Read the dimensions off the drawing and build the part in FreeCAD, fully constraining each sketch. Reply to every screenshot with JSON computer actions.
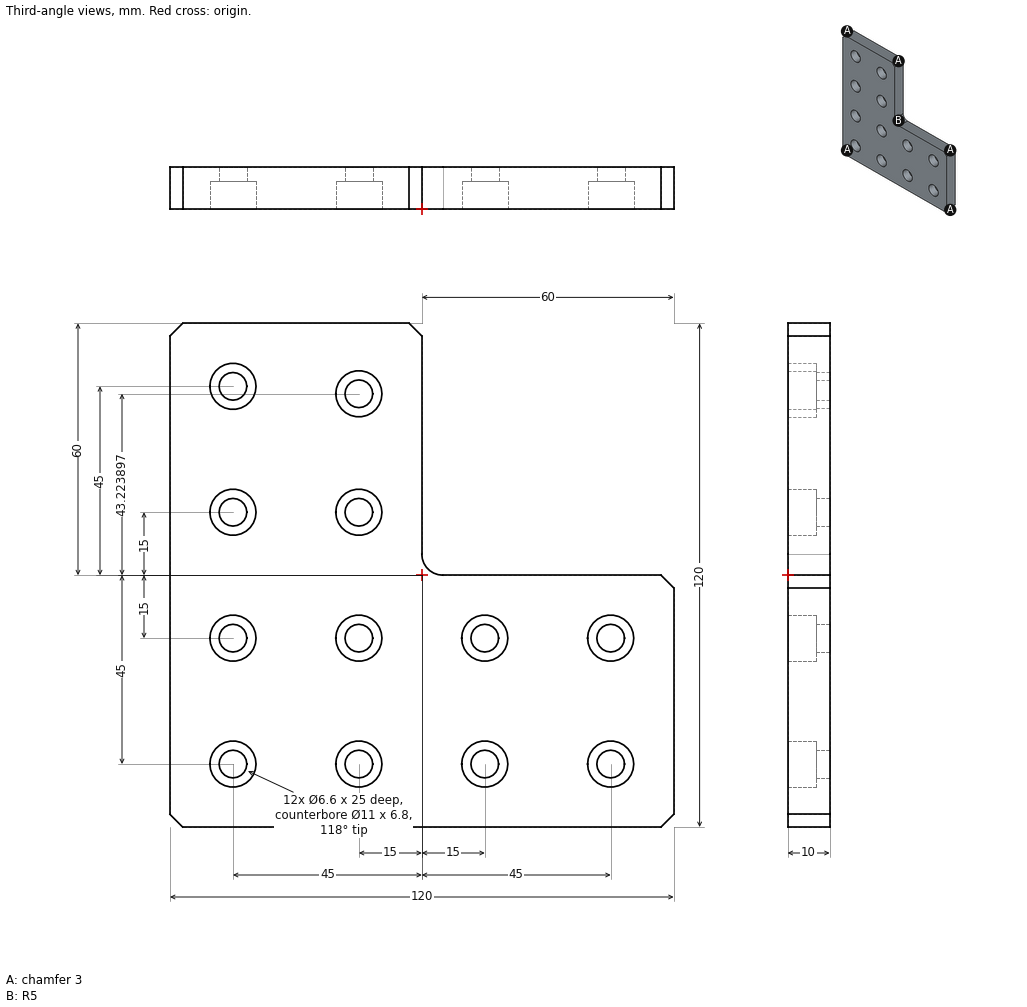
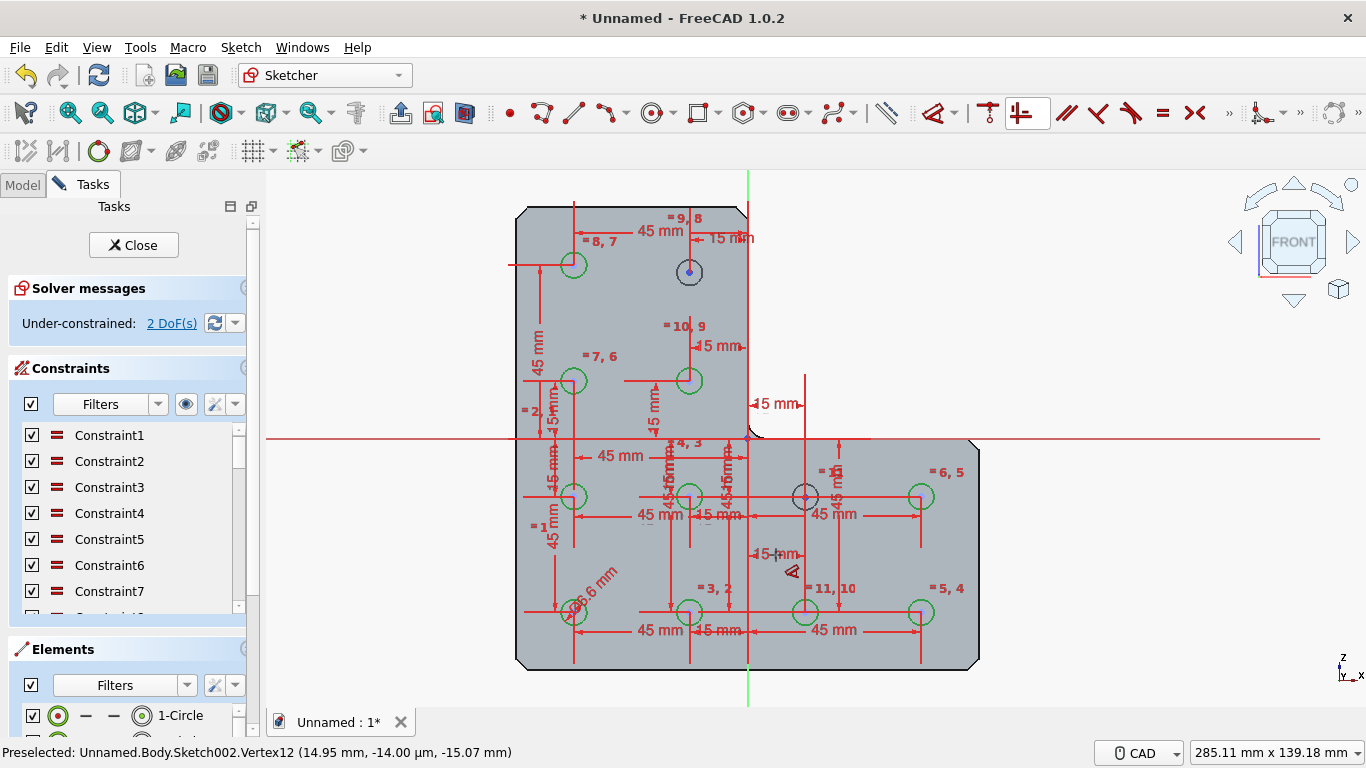
{"action": "left_click", "coordinate": [805, 497]}
{"action": "left_click", "coordinate": [839, 455]}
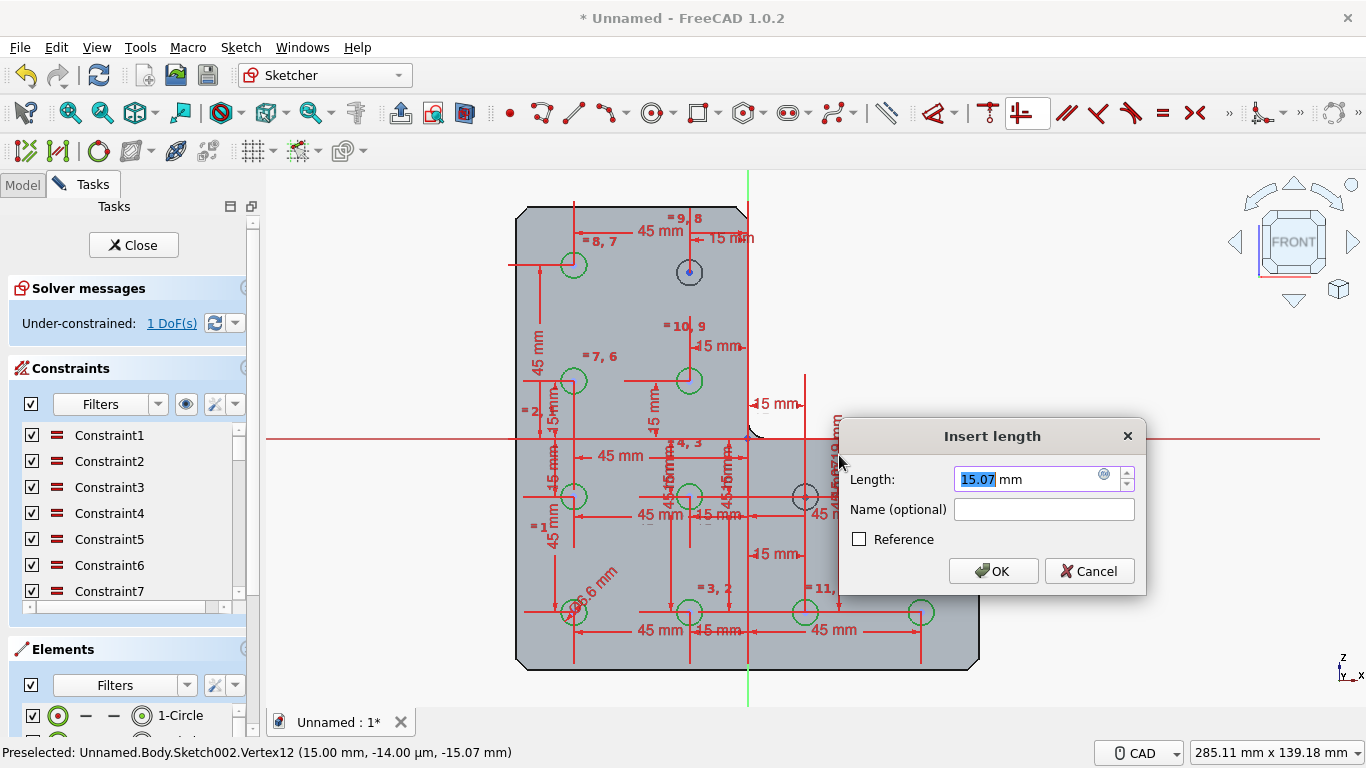
{"action": "type", "text": "15"}
{"action": "key", "text": "Return"}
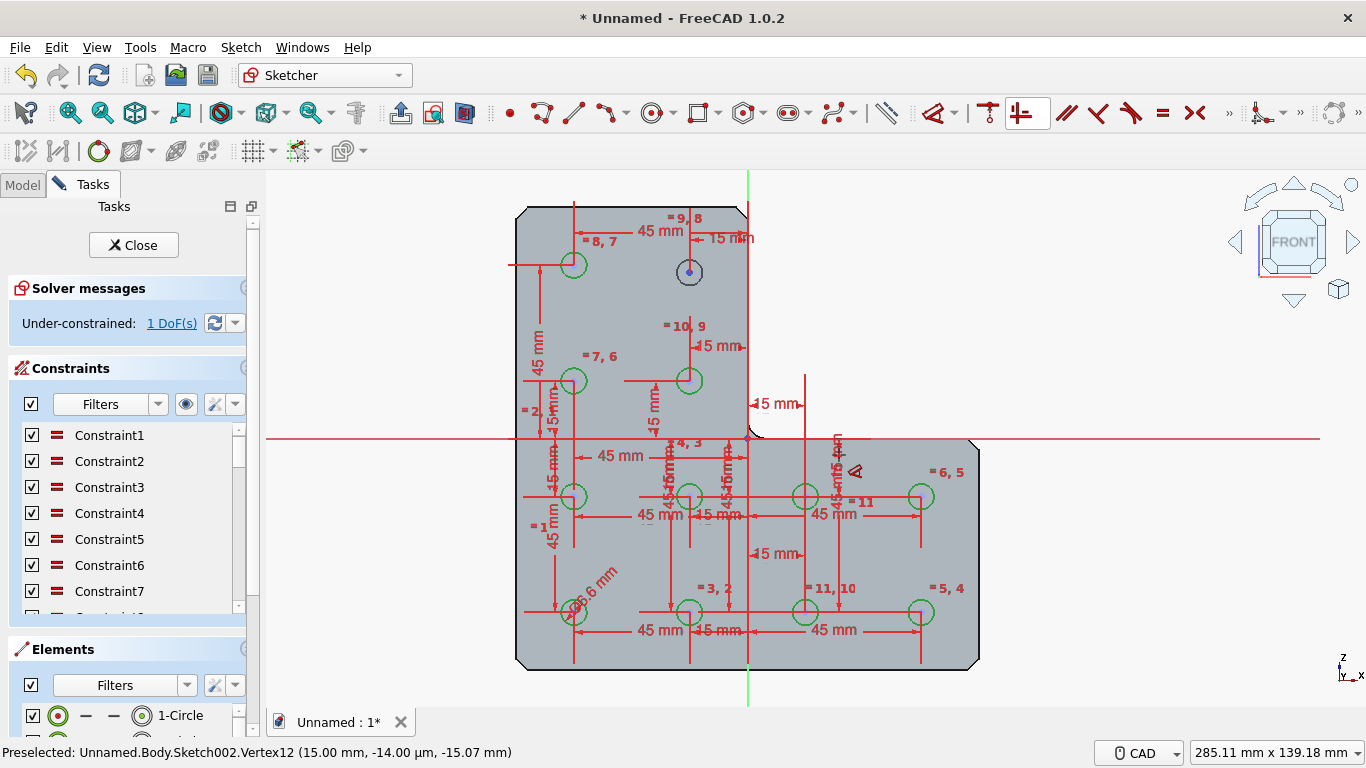
{"action": "left_click", "coordinate": [690, 273]}
{"action": "left_click", "coordinate": [656, 318]}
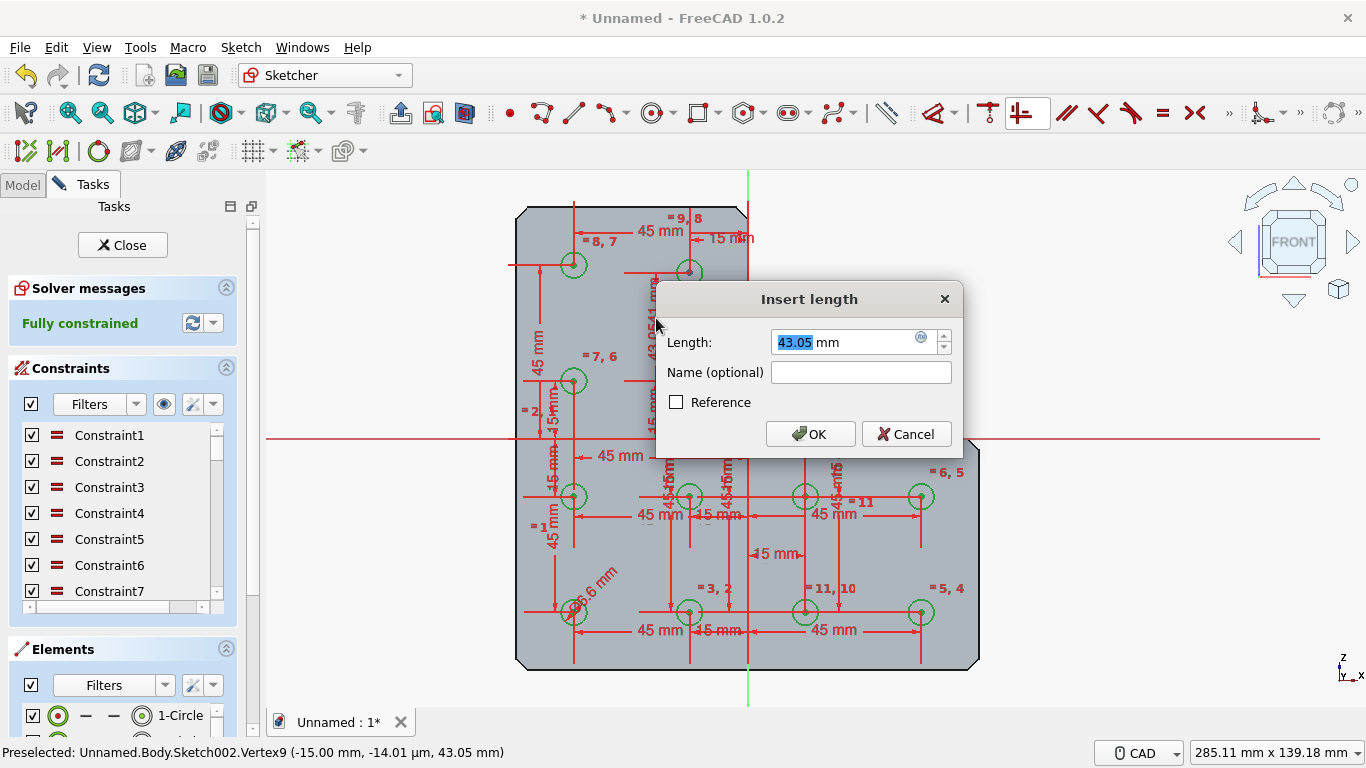
{"action": "type", "text": "43.223897"}
{"action": "key", "text": "Return"}
{"action": "key", "text": "Escape"}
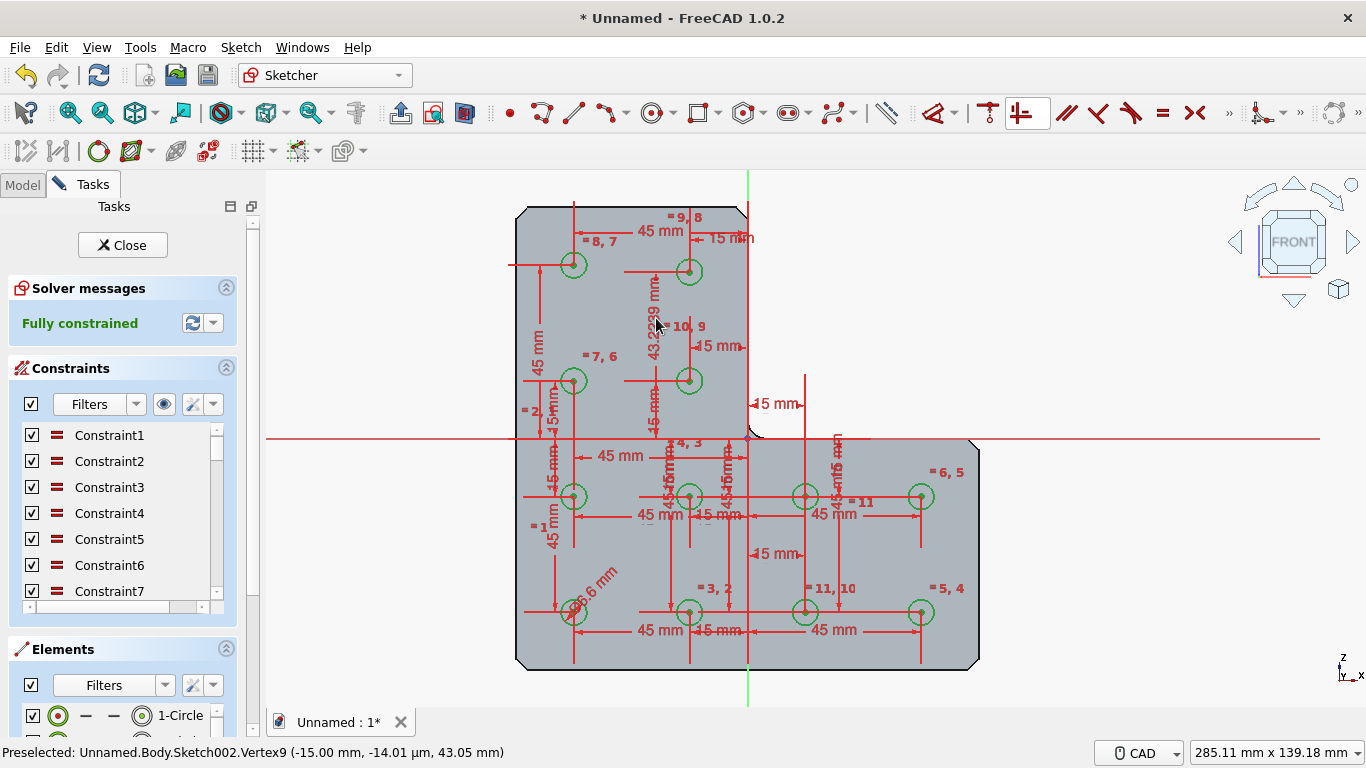
{"action": "left_click", "coordinate": [123, 245]}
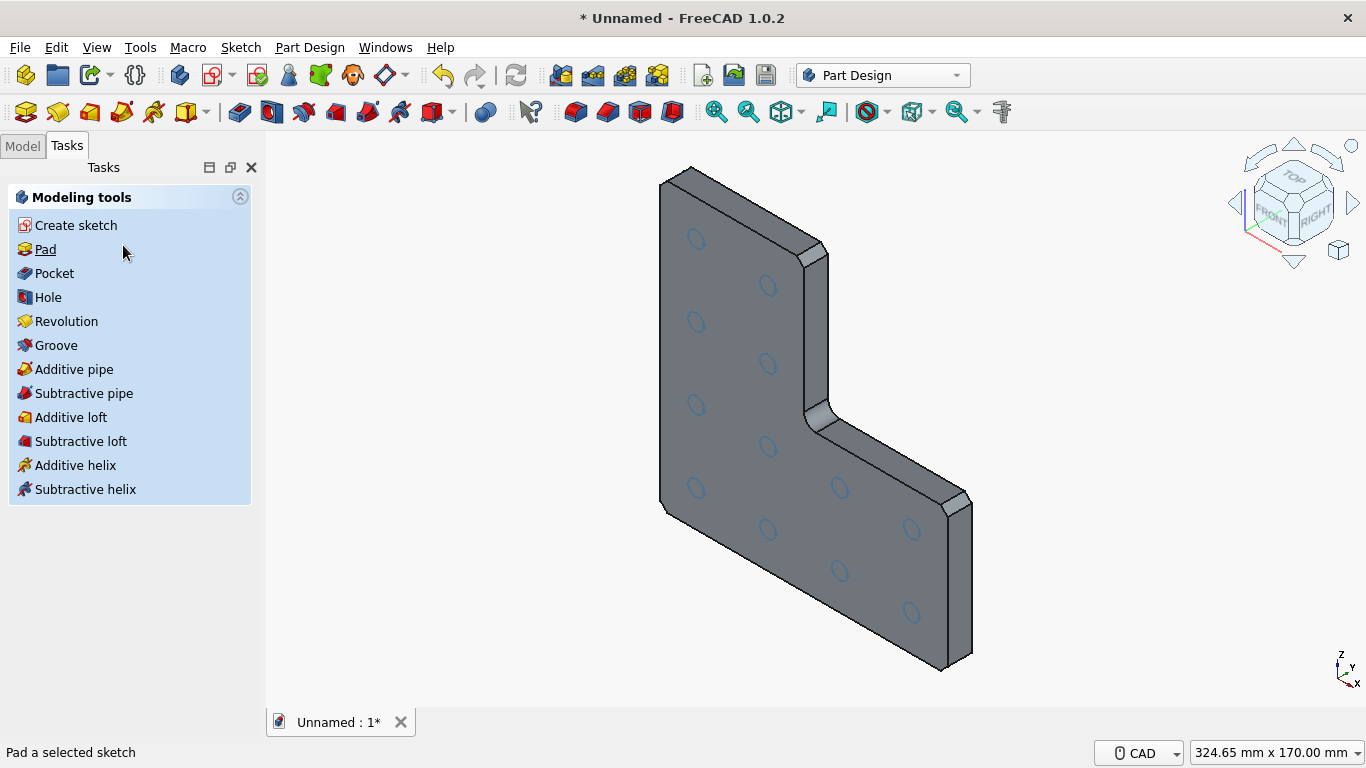
{"action": "left_click", "coordinate": [272, 112]}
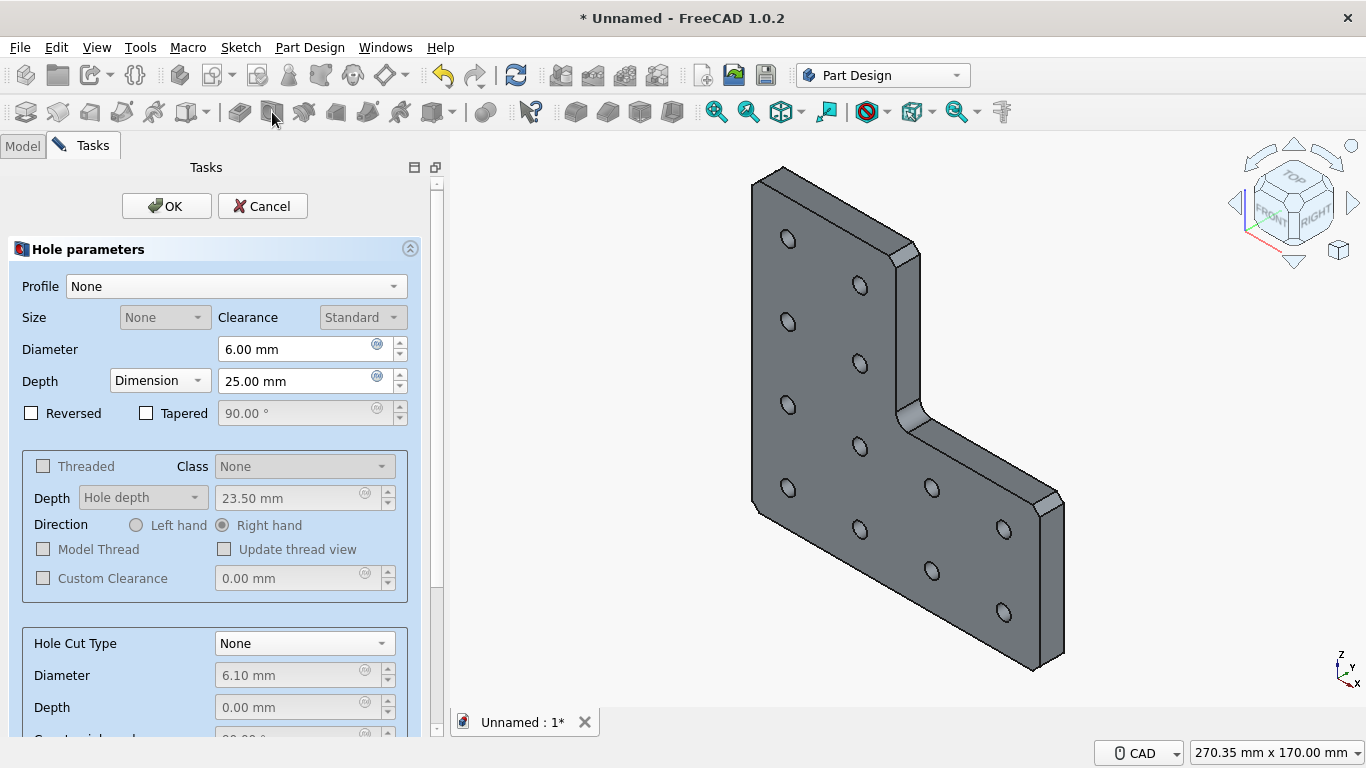
{"action": "triple_click", "coordinate": [305, 349]}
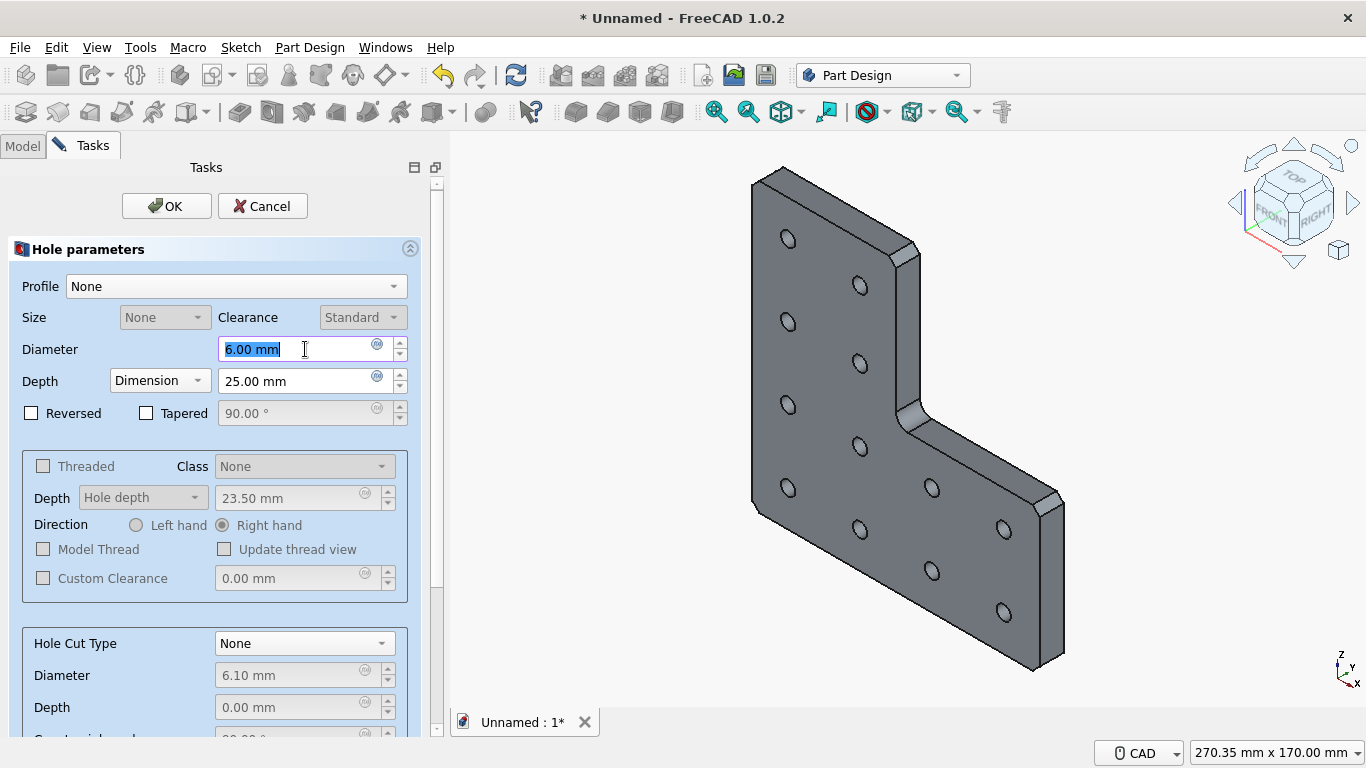
{"action": "type", "text": "6.6"}
{"action": "key", "text": "Tab"}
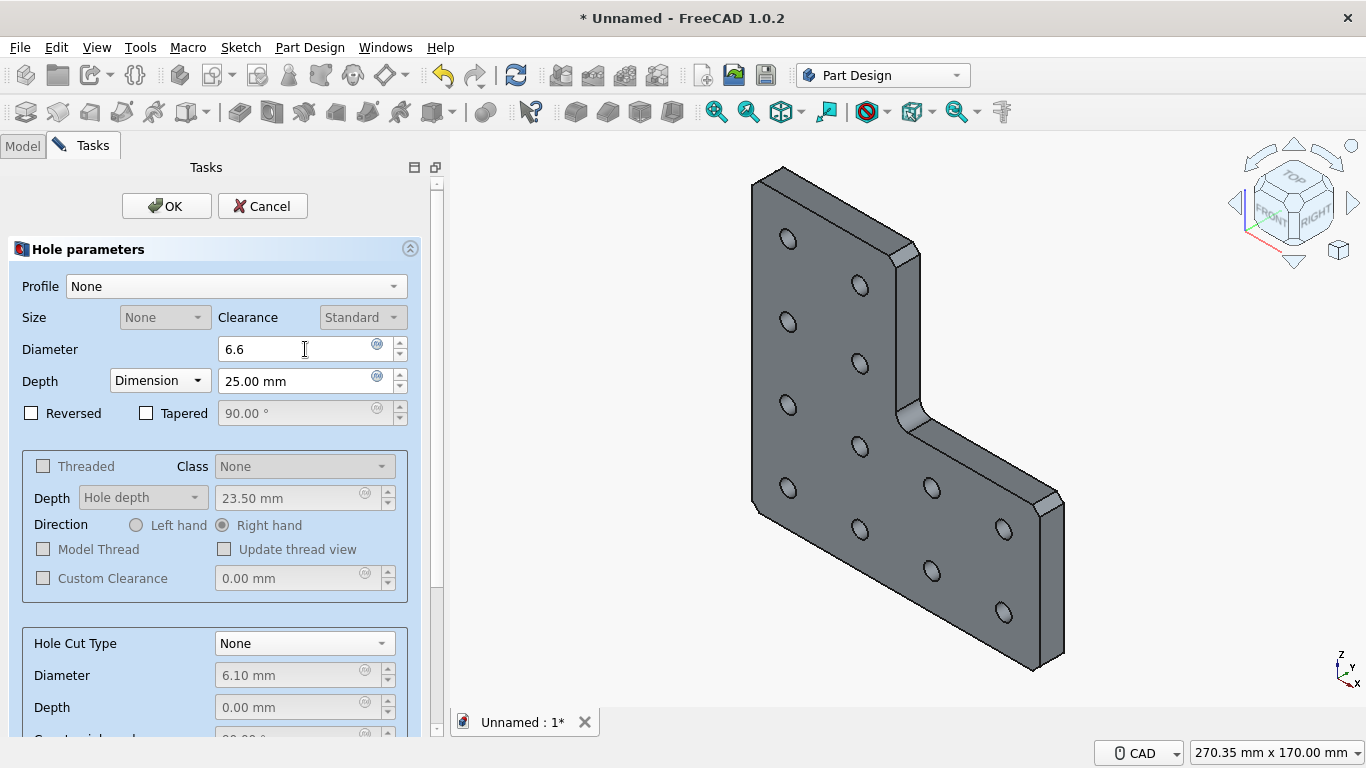
{"action": "triple_click", "coordinate": [305, 381]}